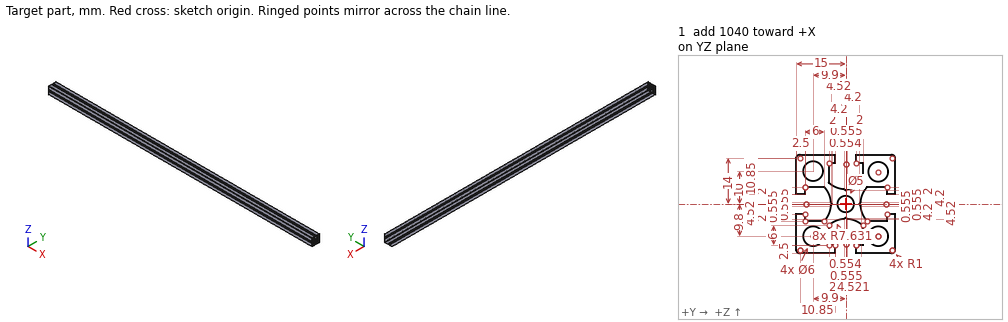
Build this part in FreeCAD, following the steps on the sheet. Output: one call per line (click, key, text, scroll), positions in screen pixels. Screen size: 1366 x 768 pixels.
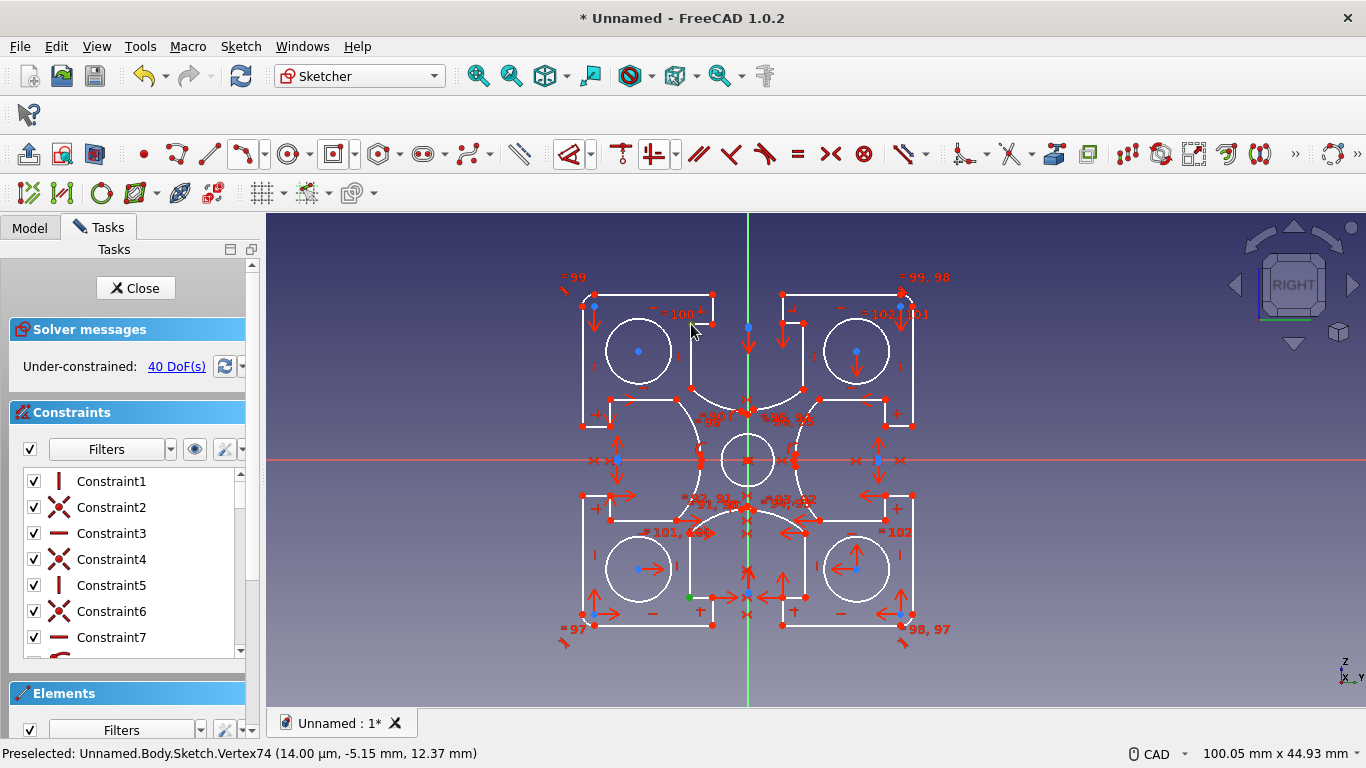
click(359, 460)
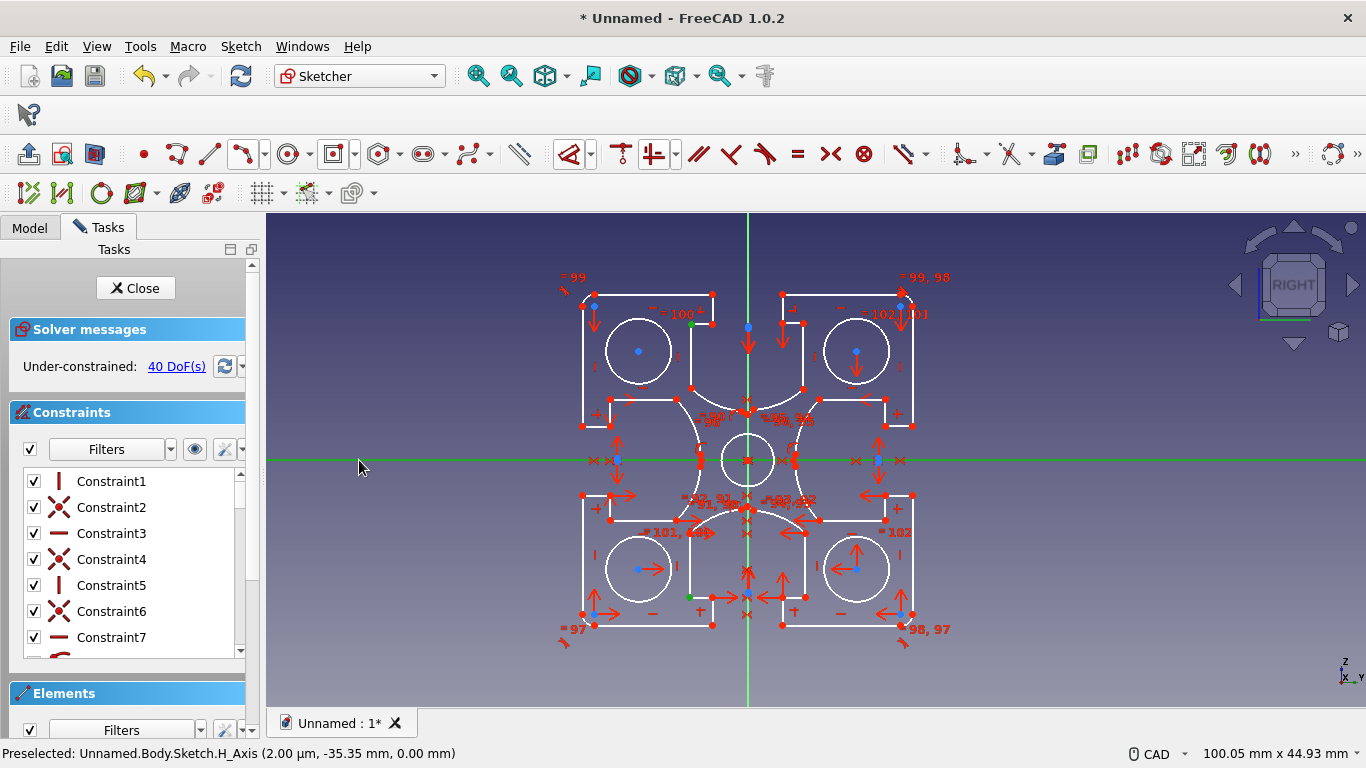
key(s)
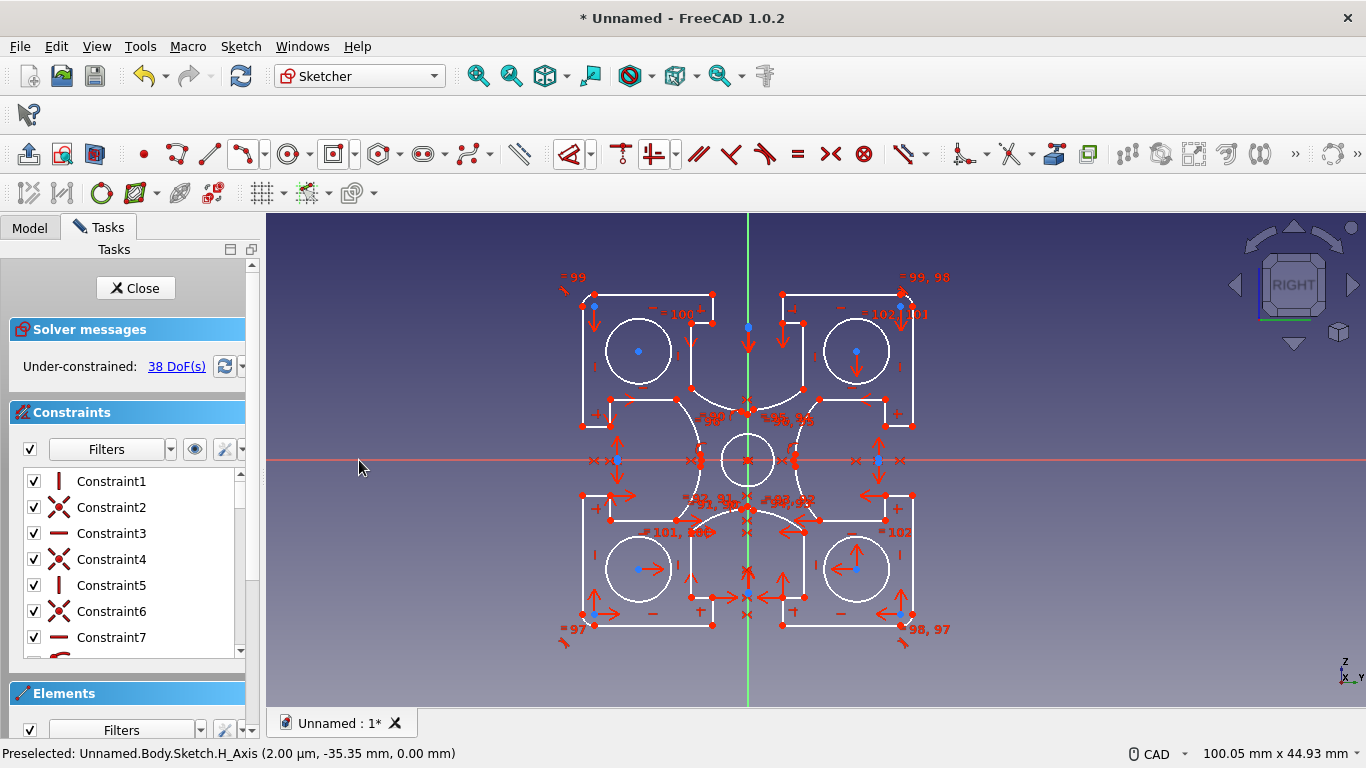
click(568, 154)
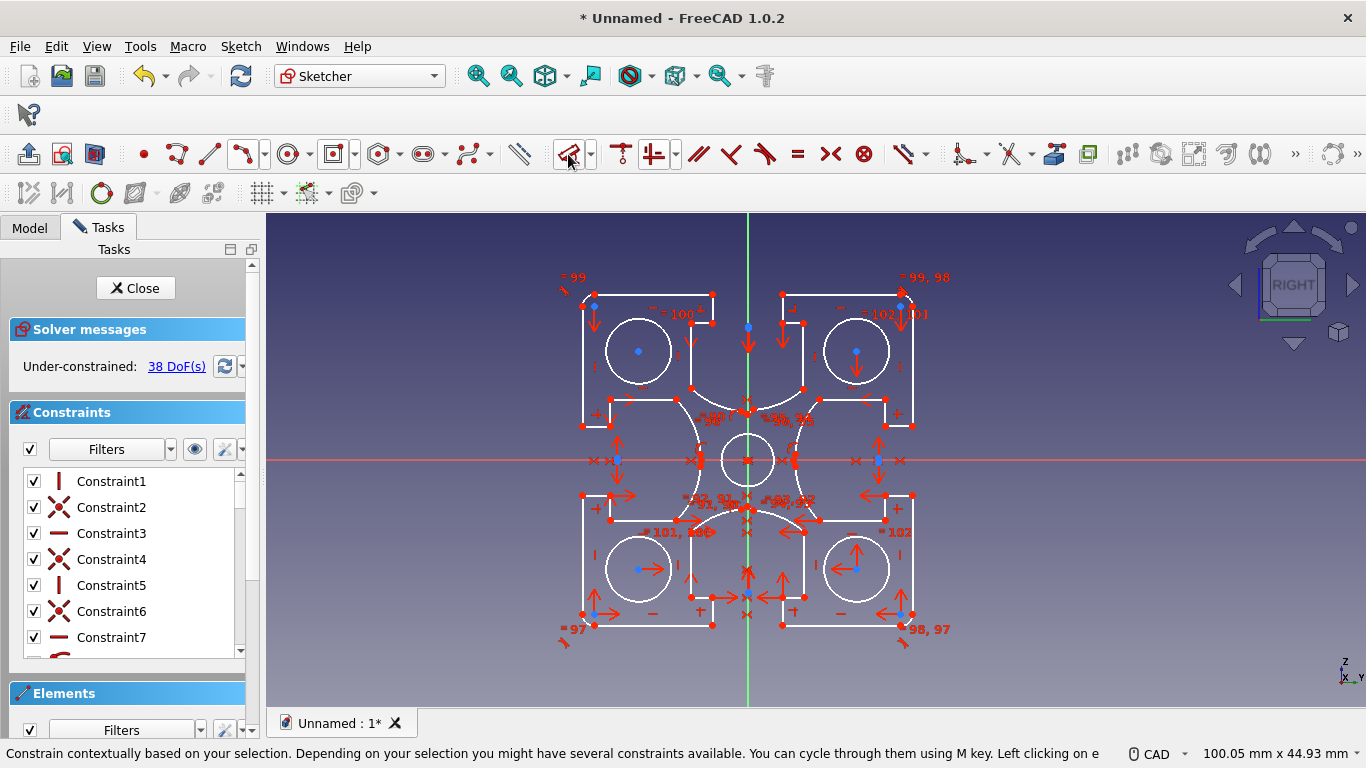
click(698, 436)
click(651, 348)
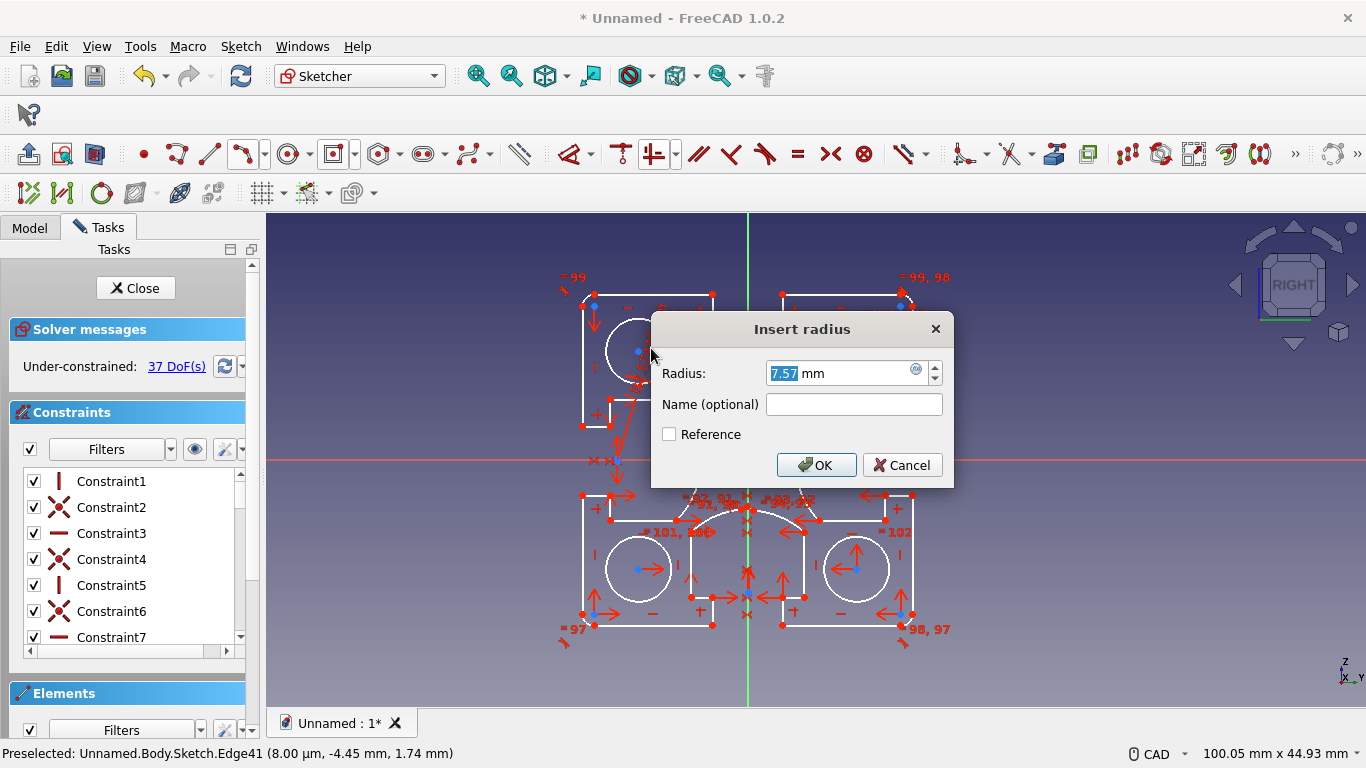
text(7.631)
key(Return)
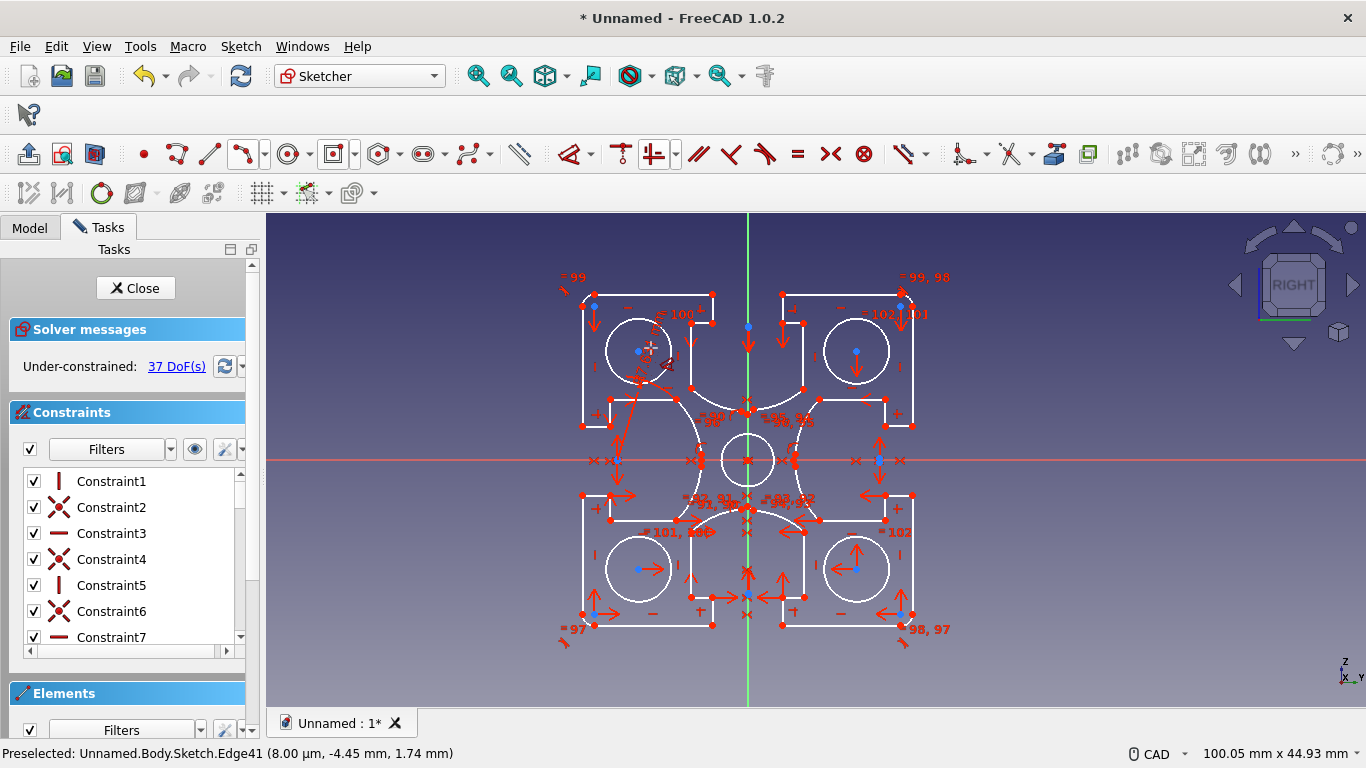
scroll(586, 622, up, 7)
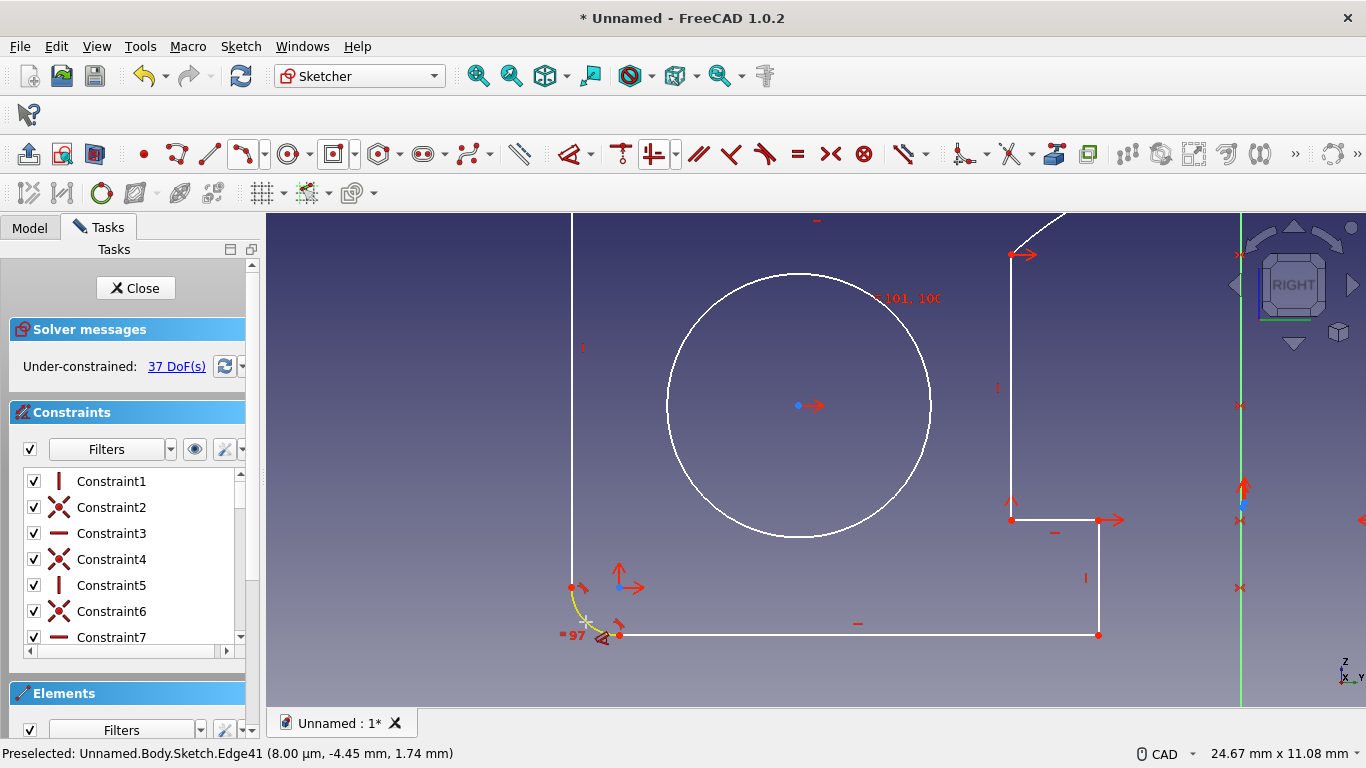
click(586, 621)
click(563, 644)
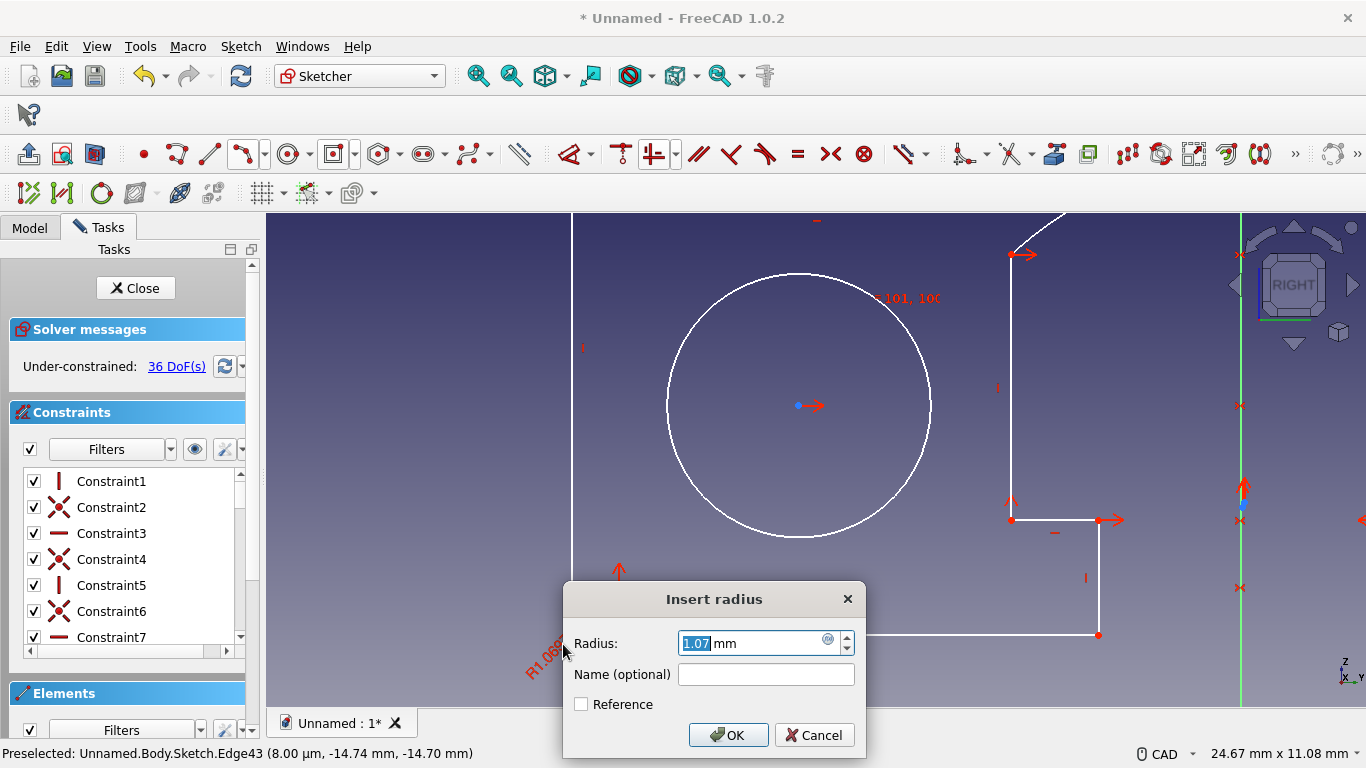
text(1)
key(Return)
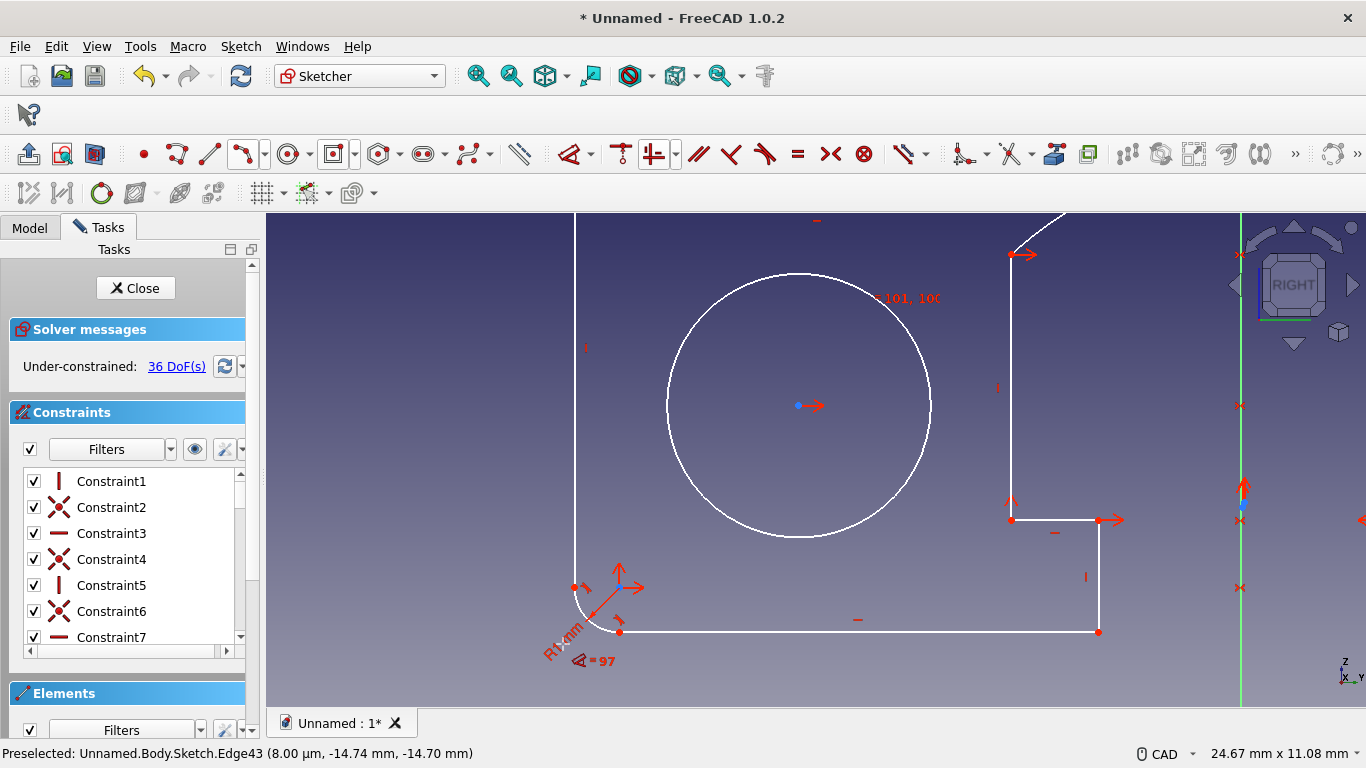
scroll(586, 622, down, 7)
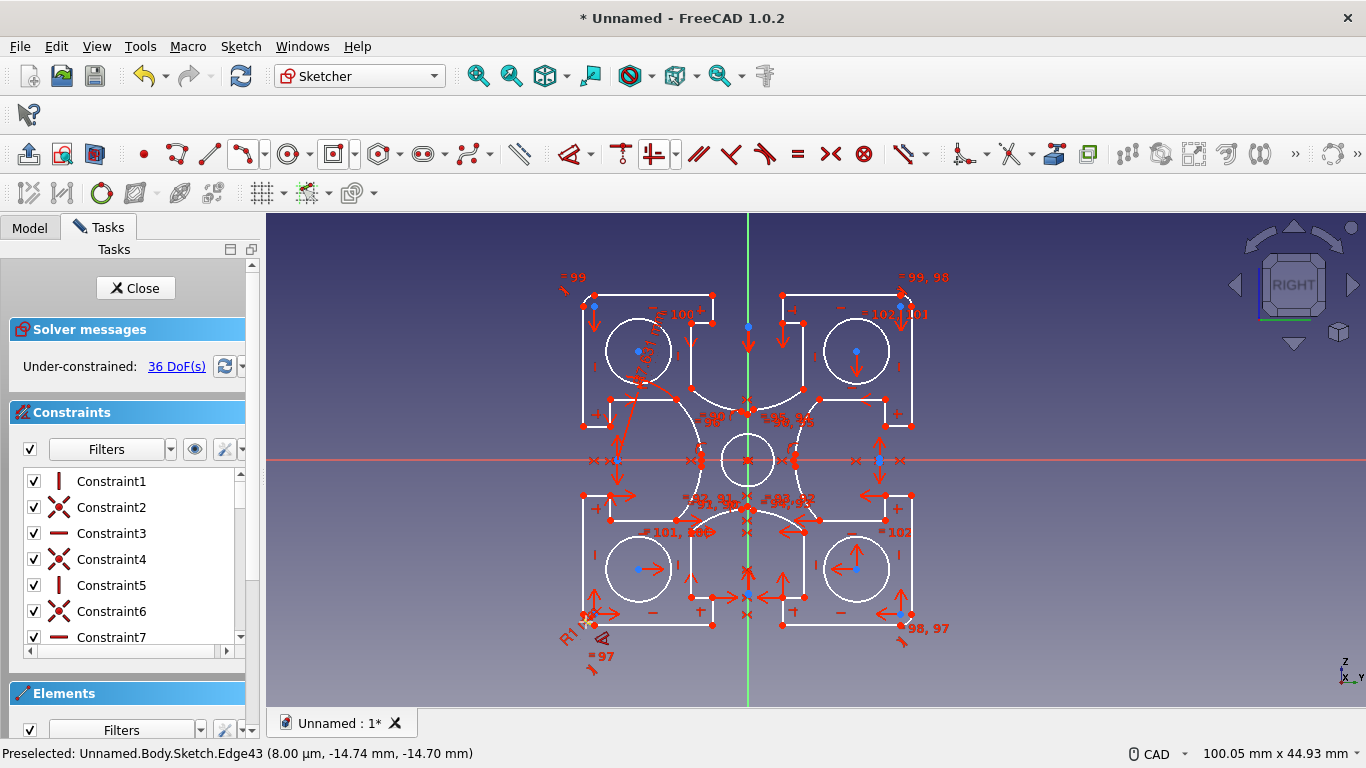
click(662, 328)
click(663, 267)